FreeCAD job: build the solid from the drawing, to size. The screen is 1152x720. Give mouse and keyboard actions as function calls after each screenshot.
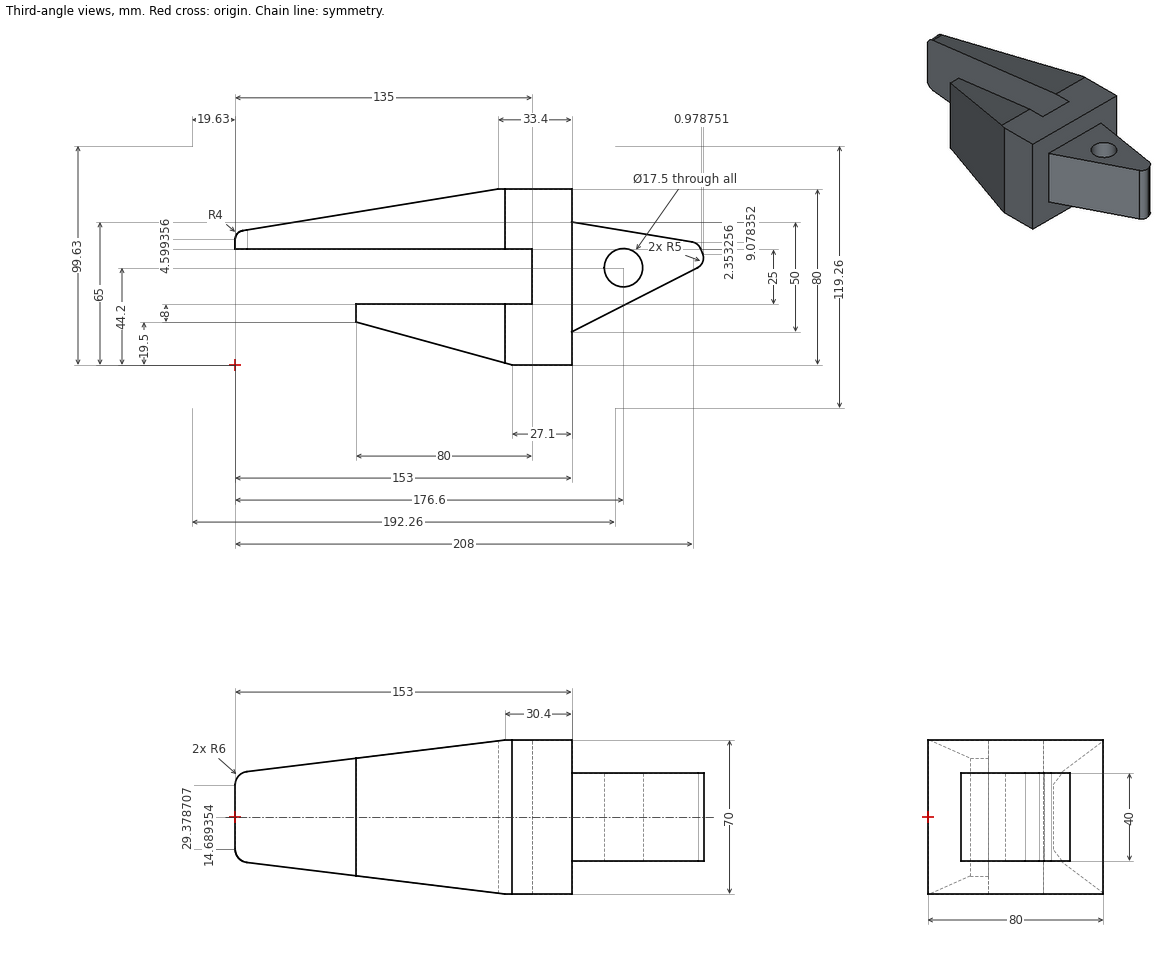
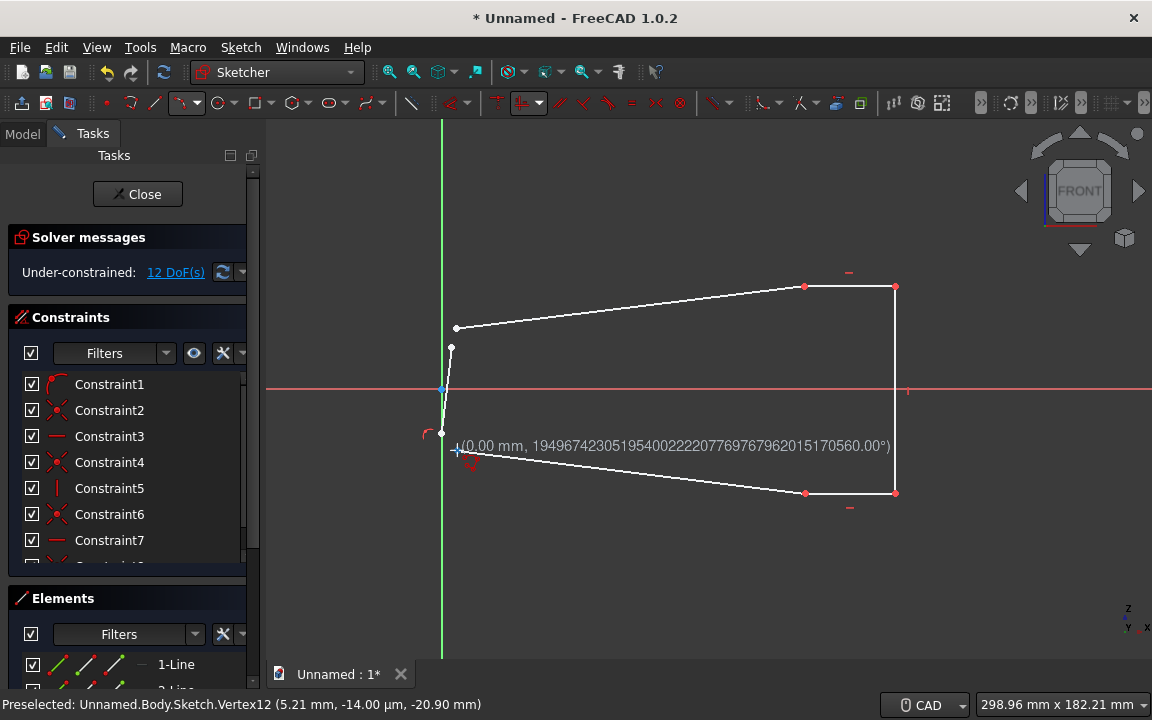
click(180, 104)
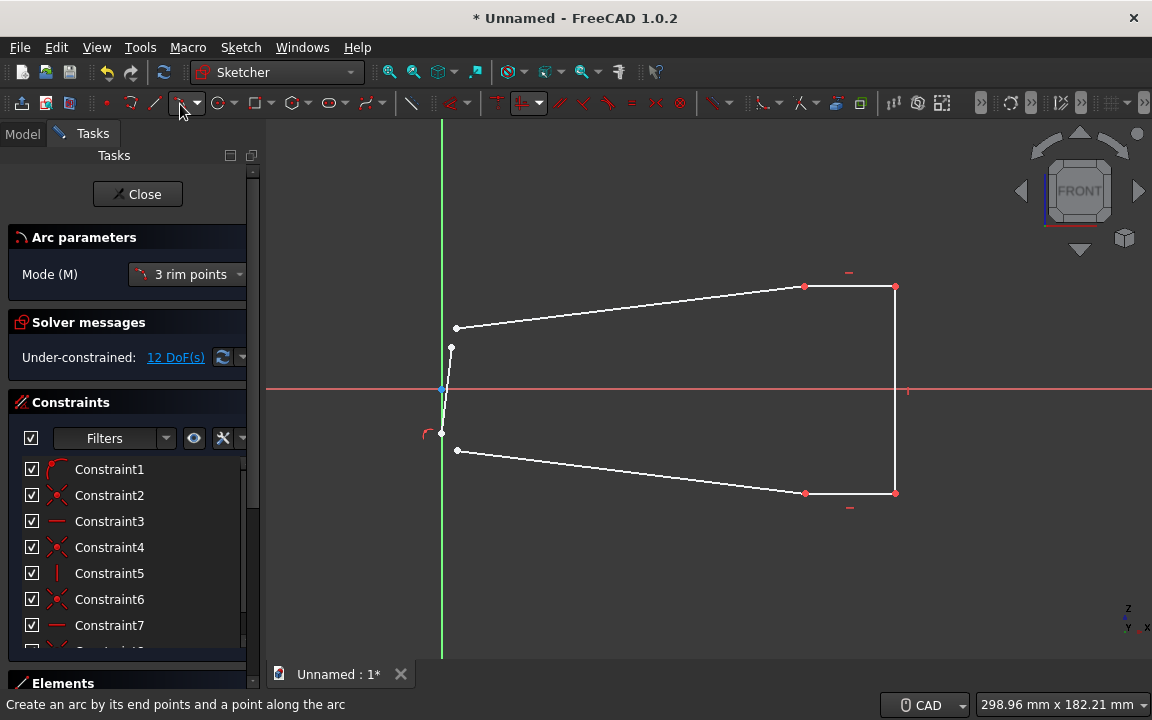
click(452, 347)
click(457, 329)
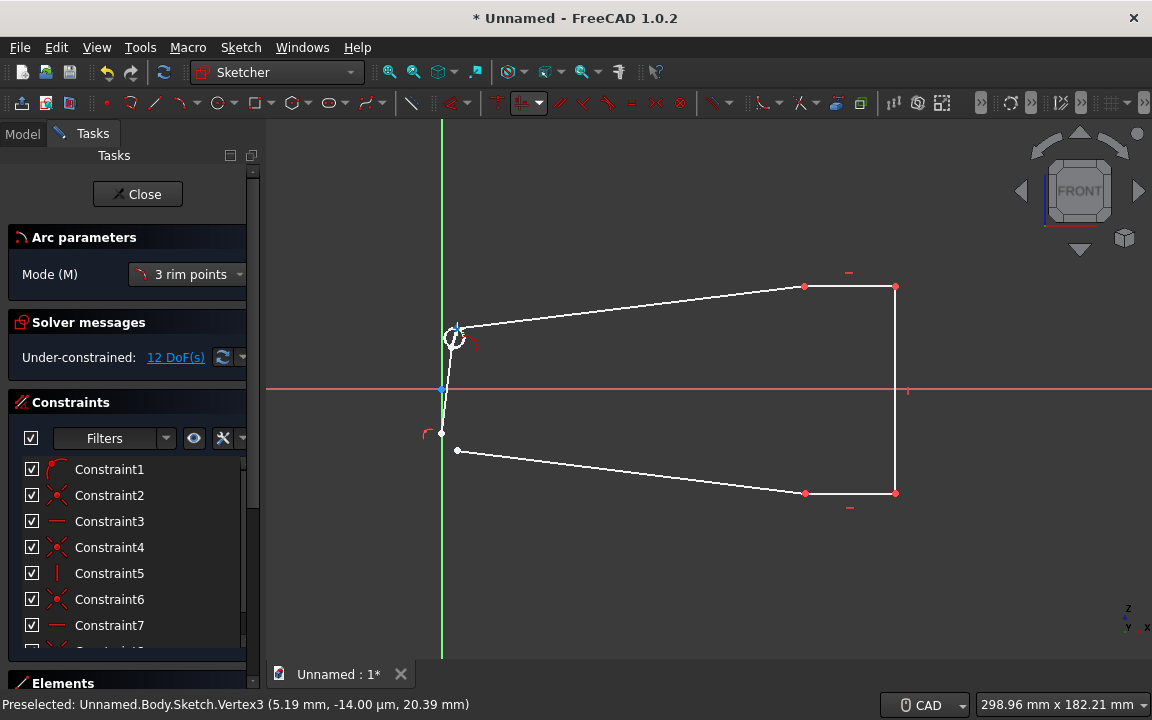
scroll(446, 334, up, 7)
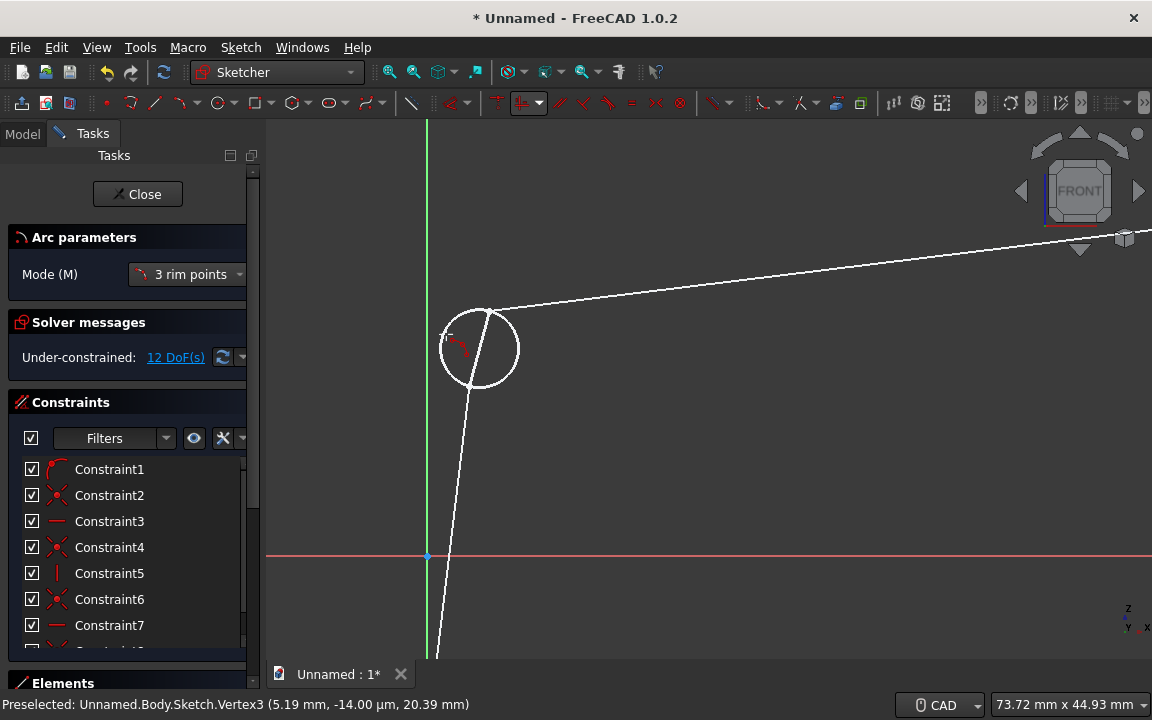
click(445, 332)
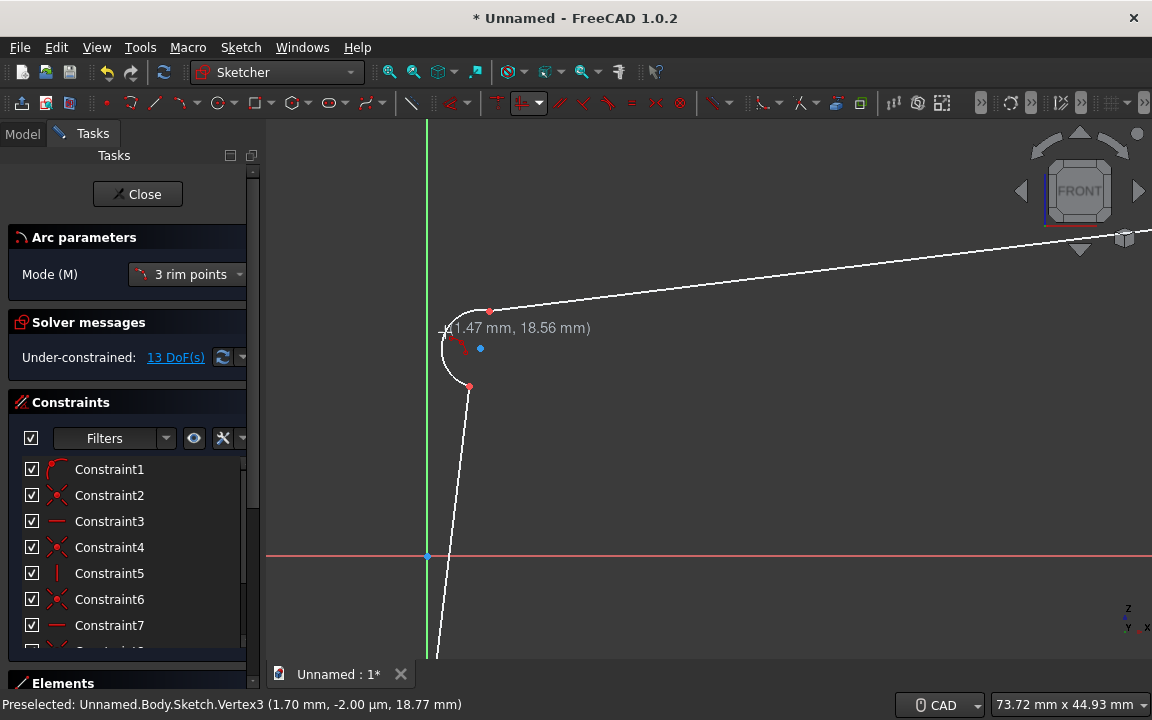
scroll(409, 334, down, 7)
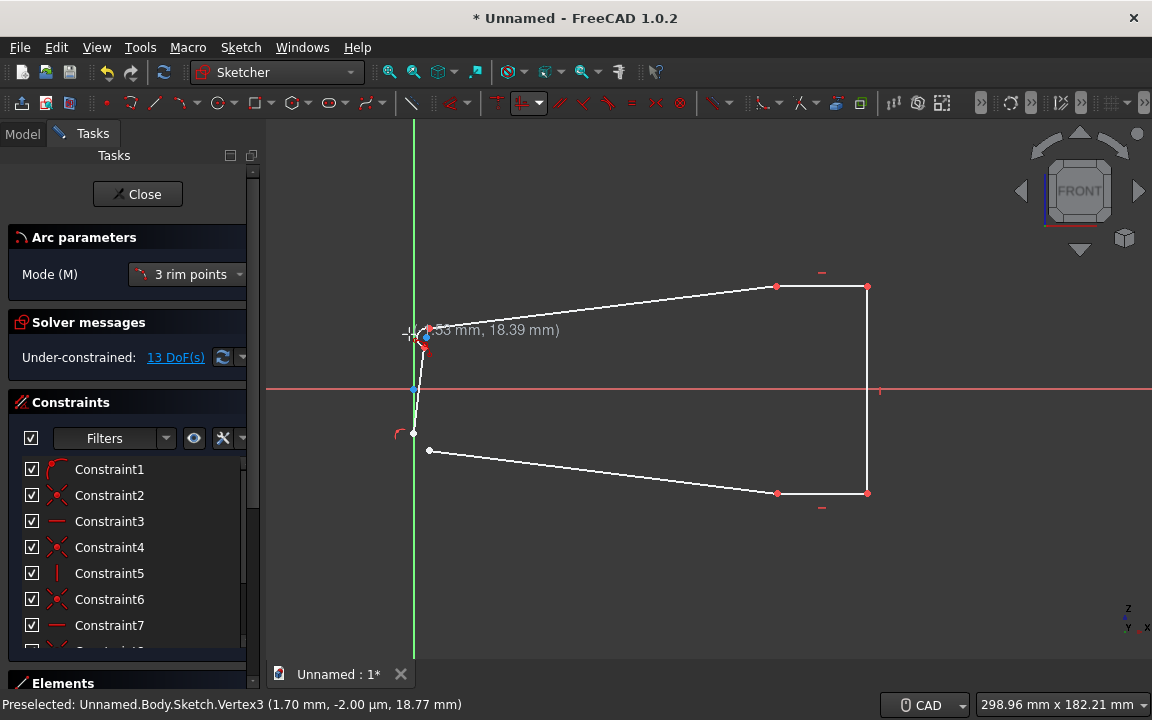
click(429, 451)
click(414, 434)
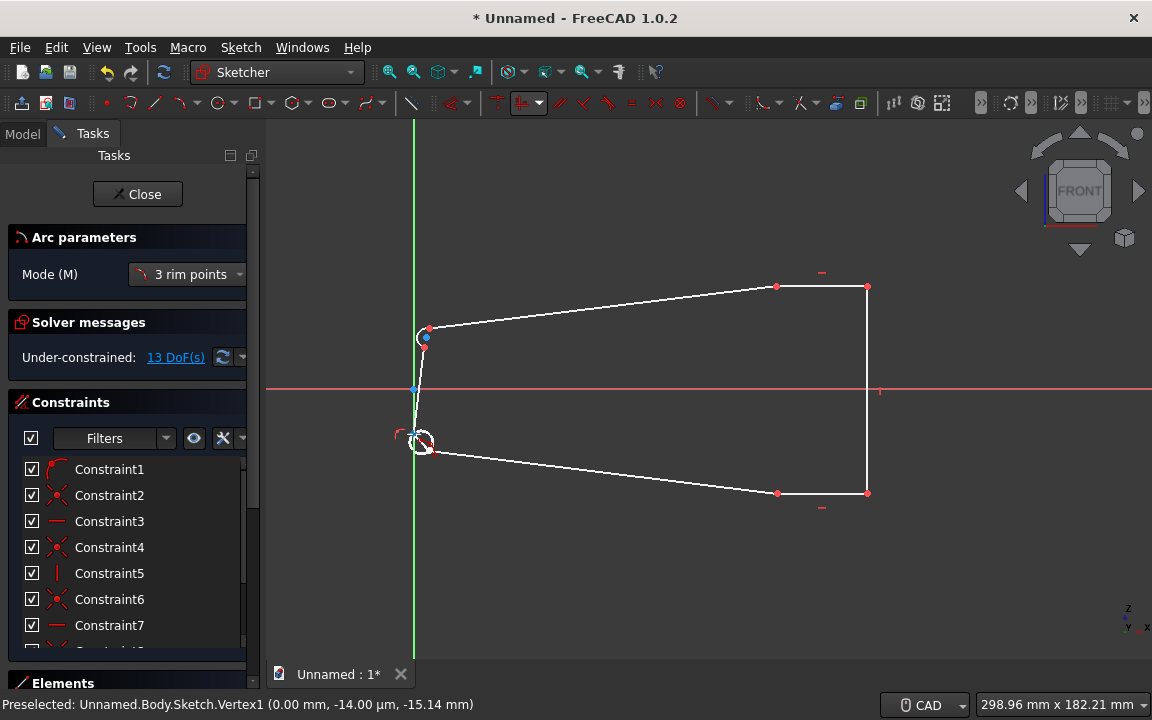
scroll(418, 444, up, 7)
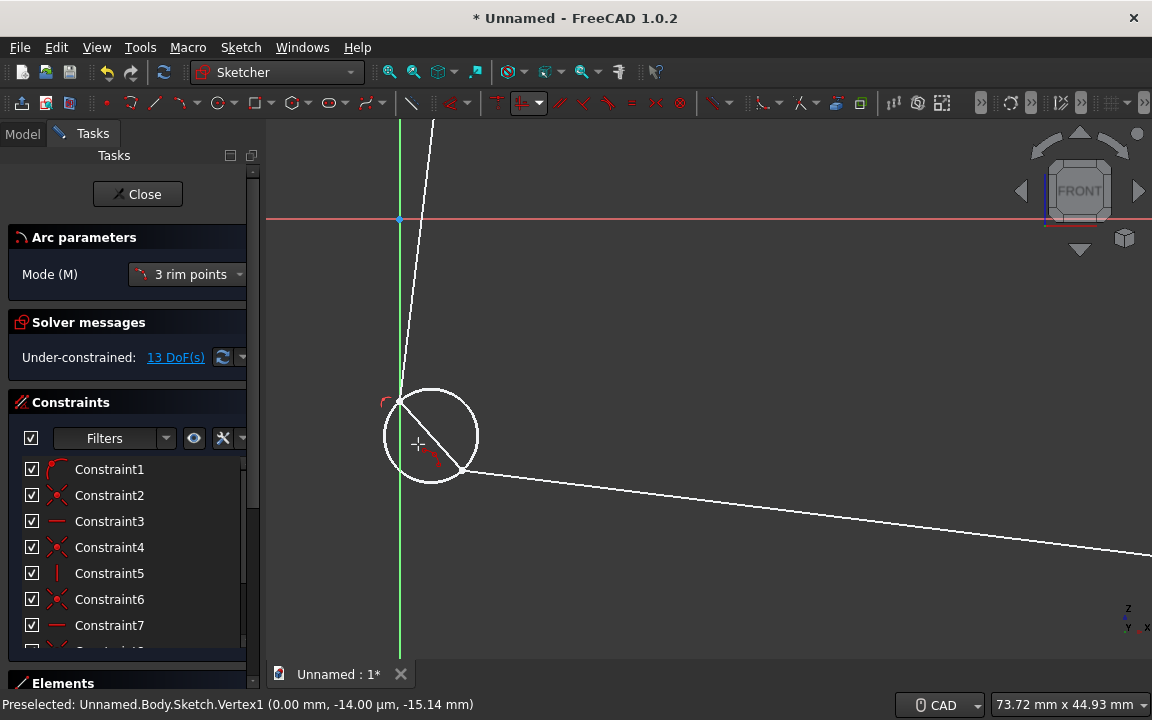
click(418, 444)
key(Escape)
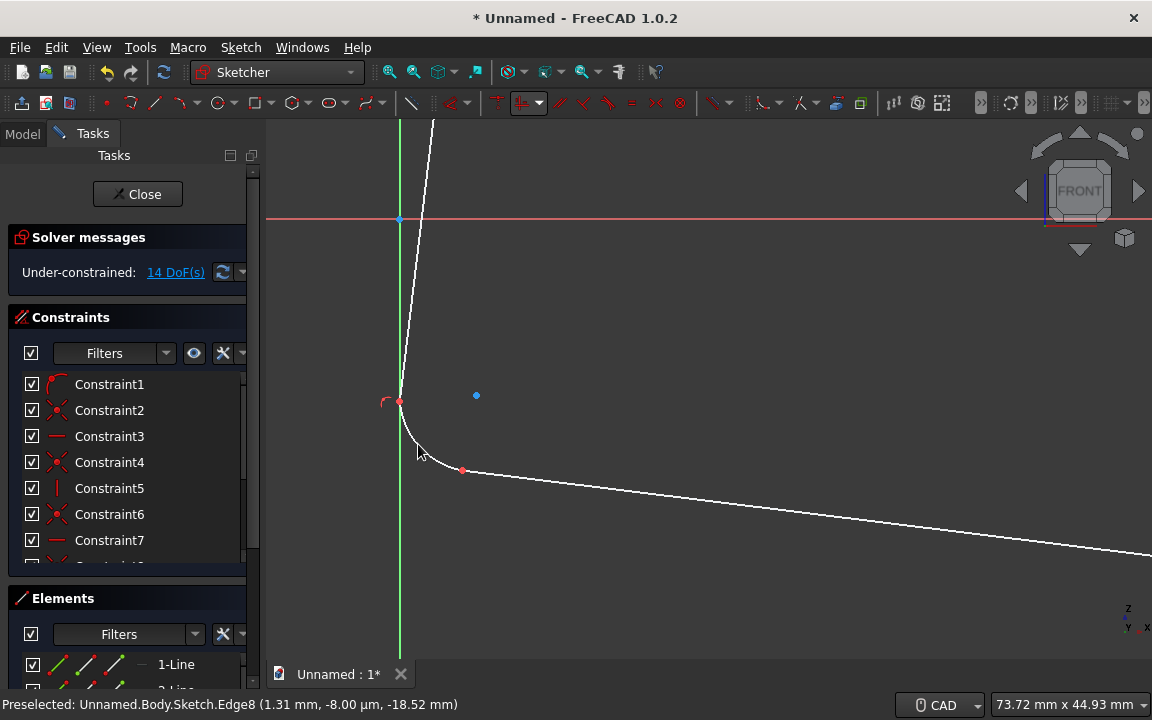
click(412, 296)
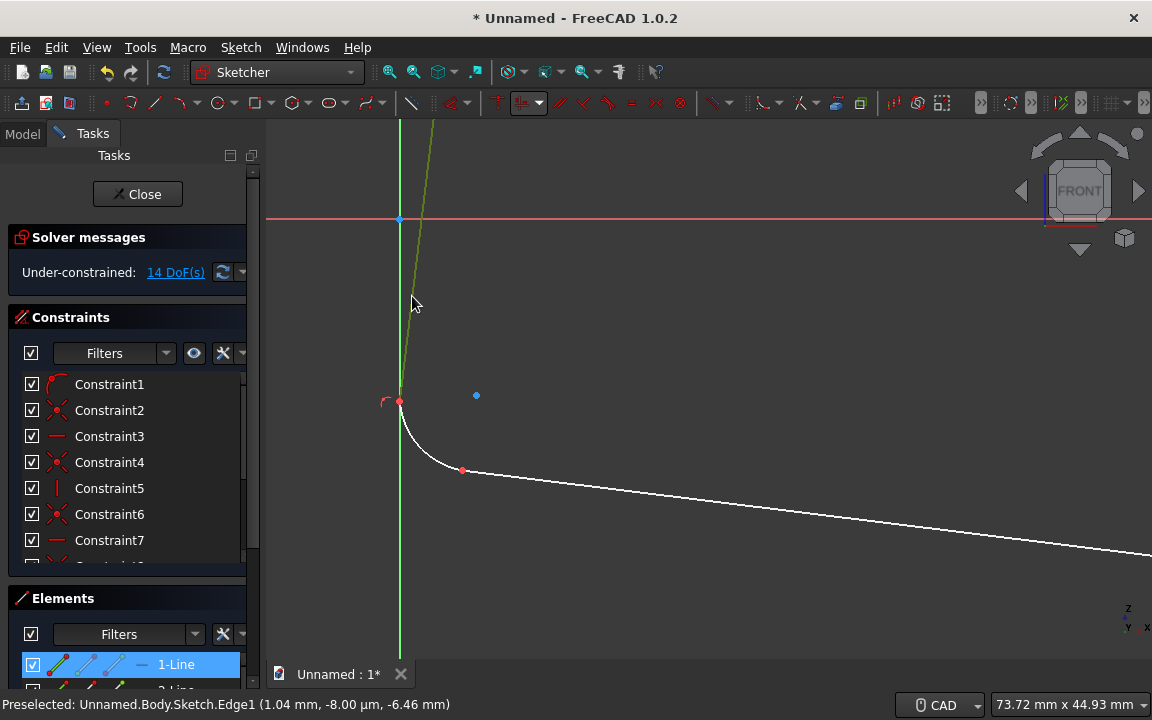
scroll(418, 445, down, 7)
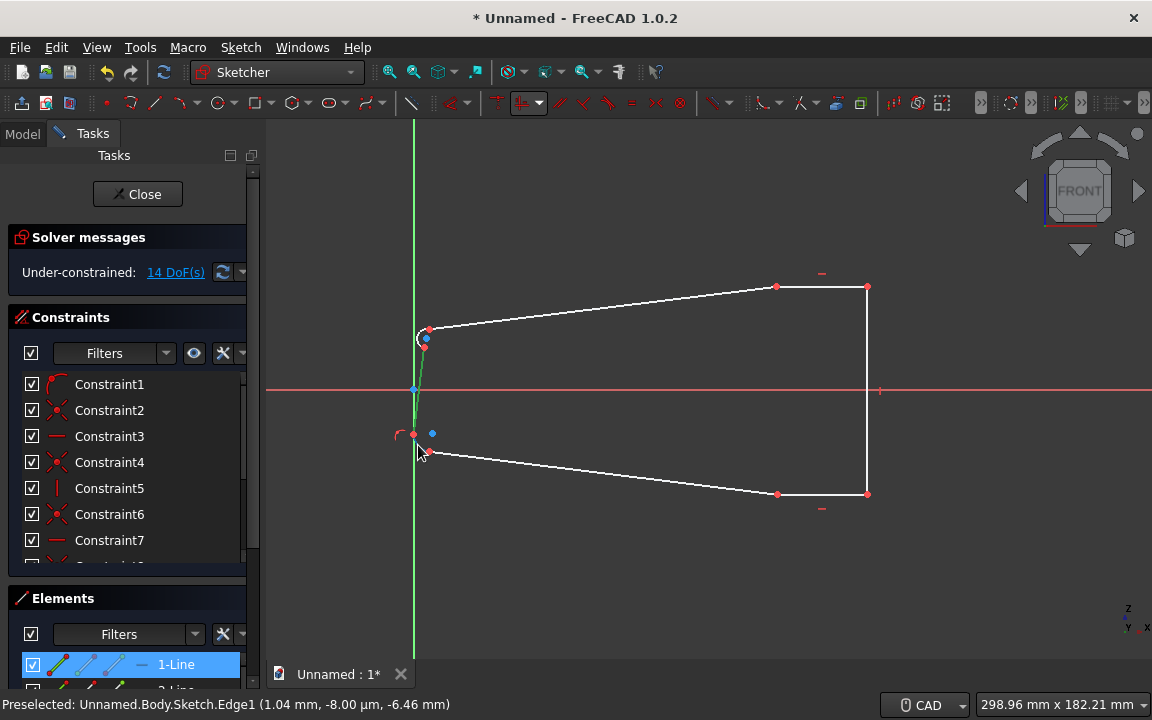
scroll(421, 331, up, 4)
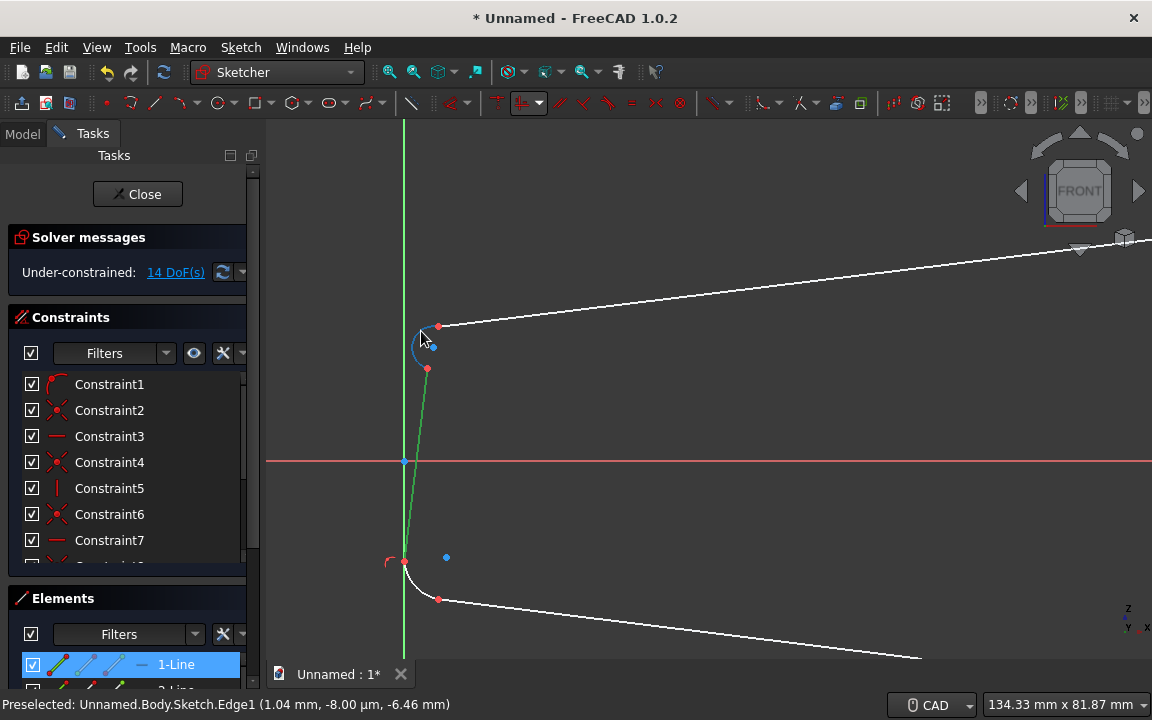
click(420, 331)